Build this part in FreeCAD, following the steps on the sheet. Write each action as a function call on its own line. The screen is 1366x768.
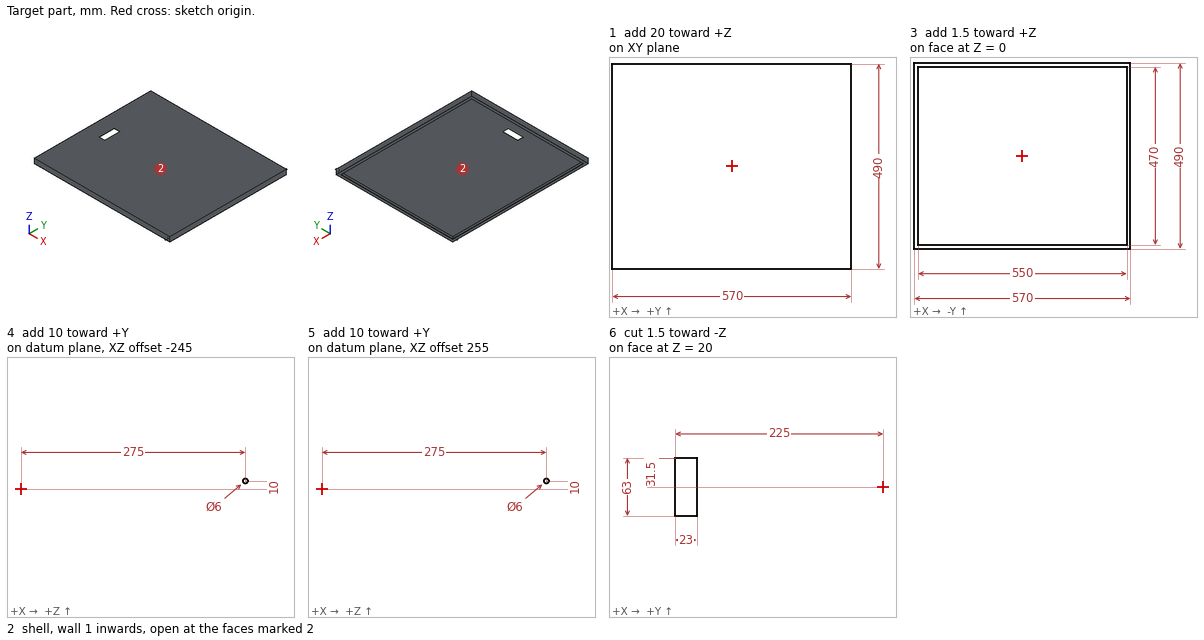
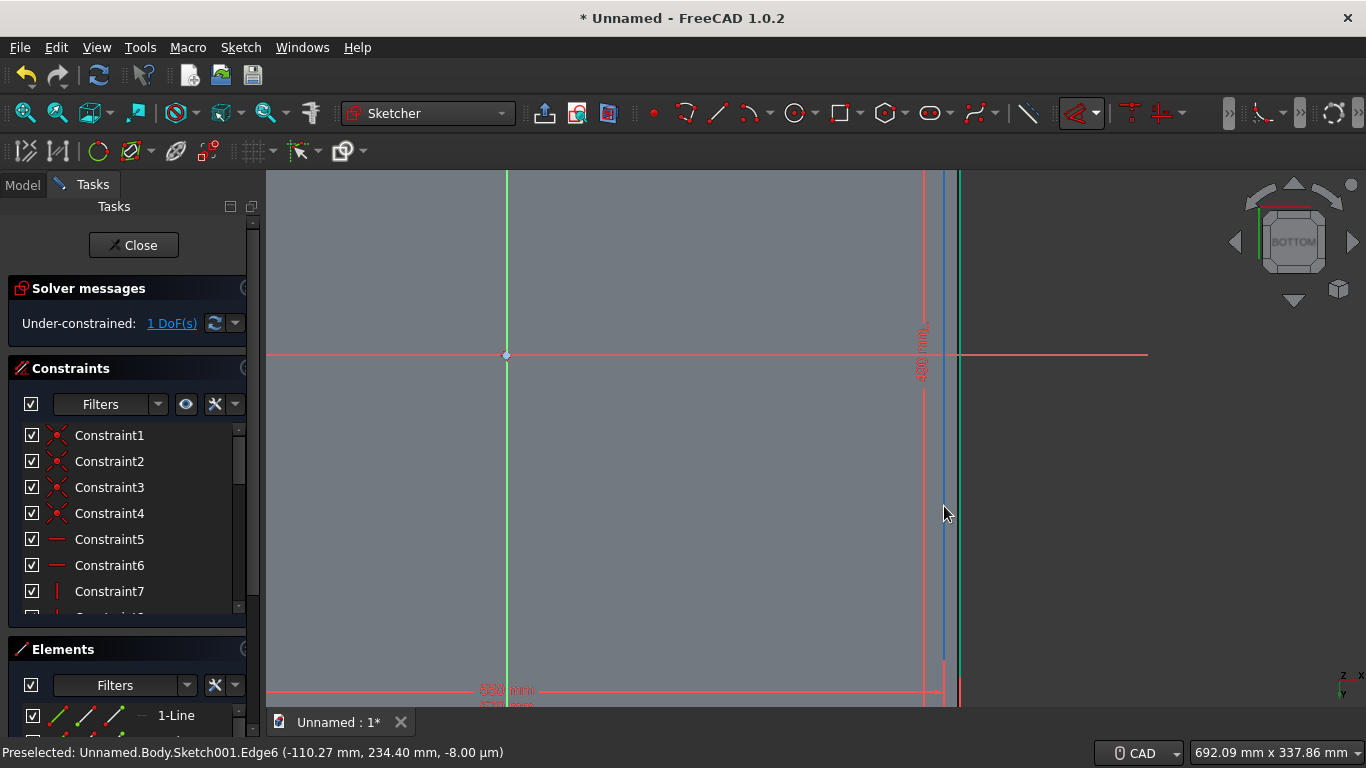
click(944, 504)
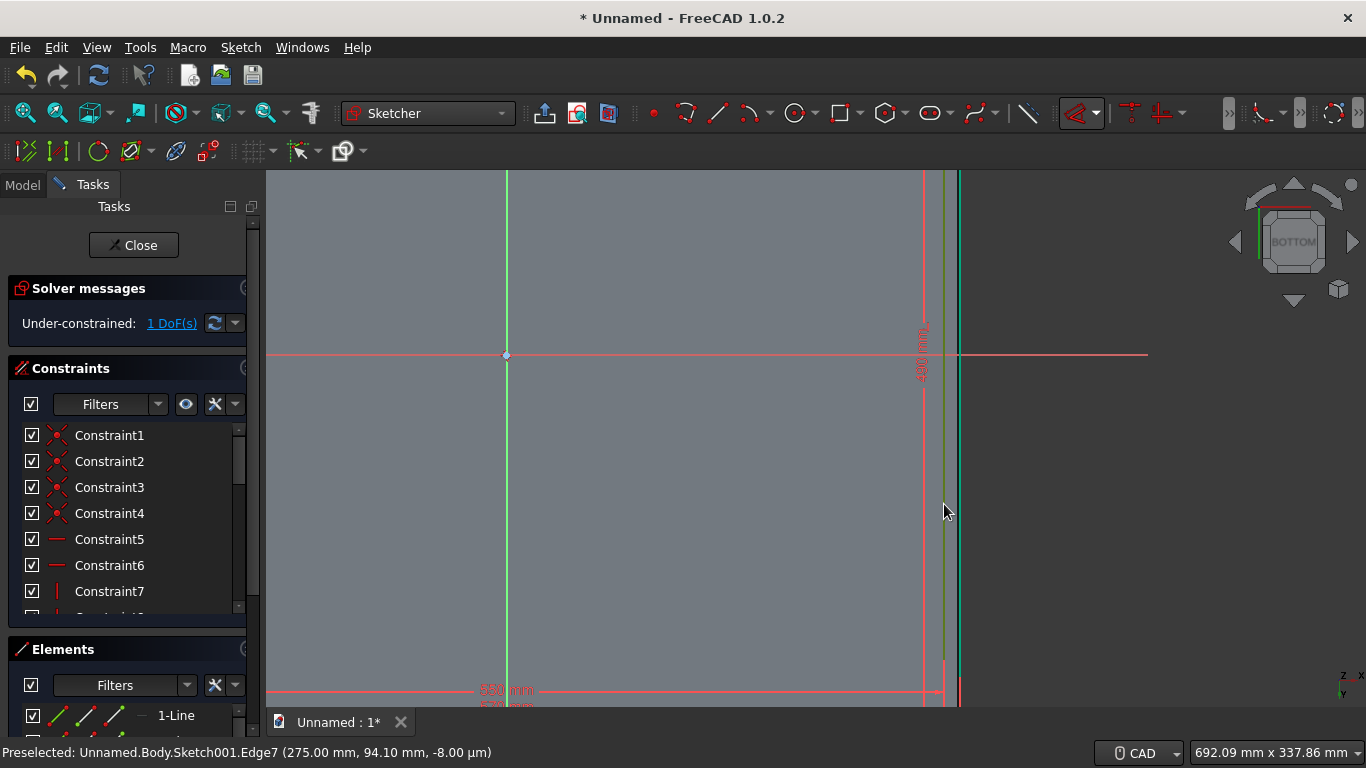
click(1098, 114)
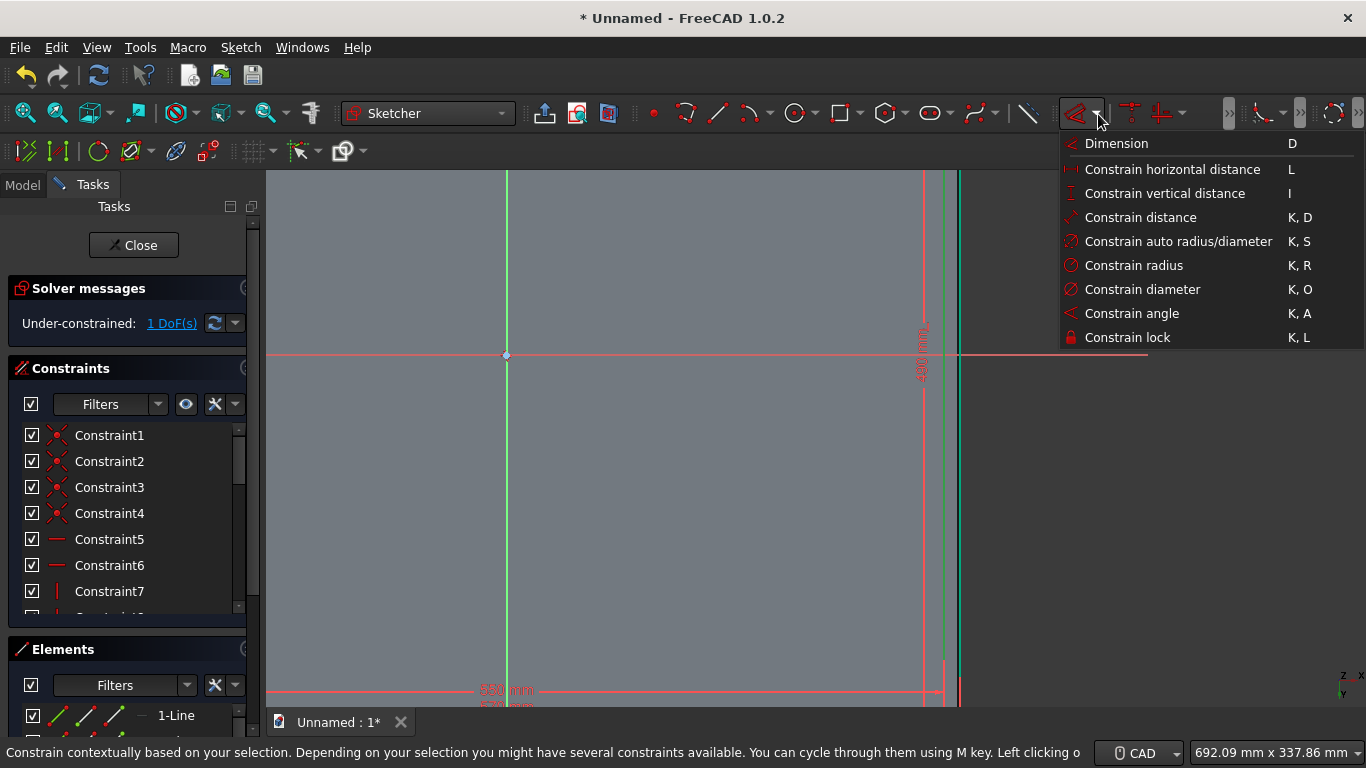
click(1212, 193)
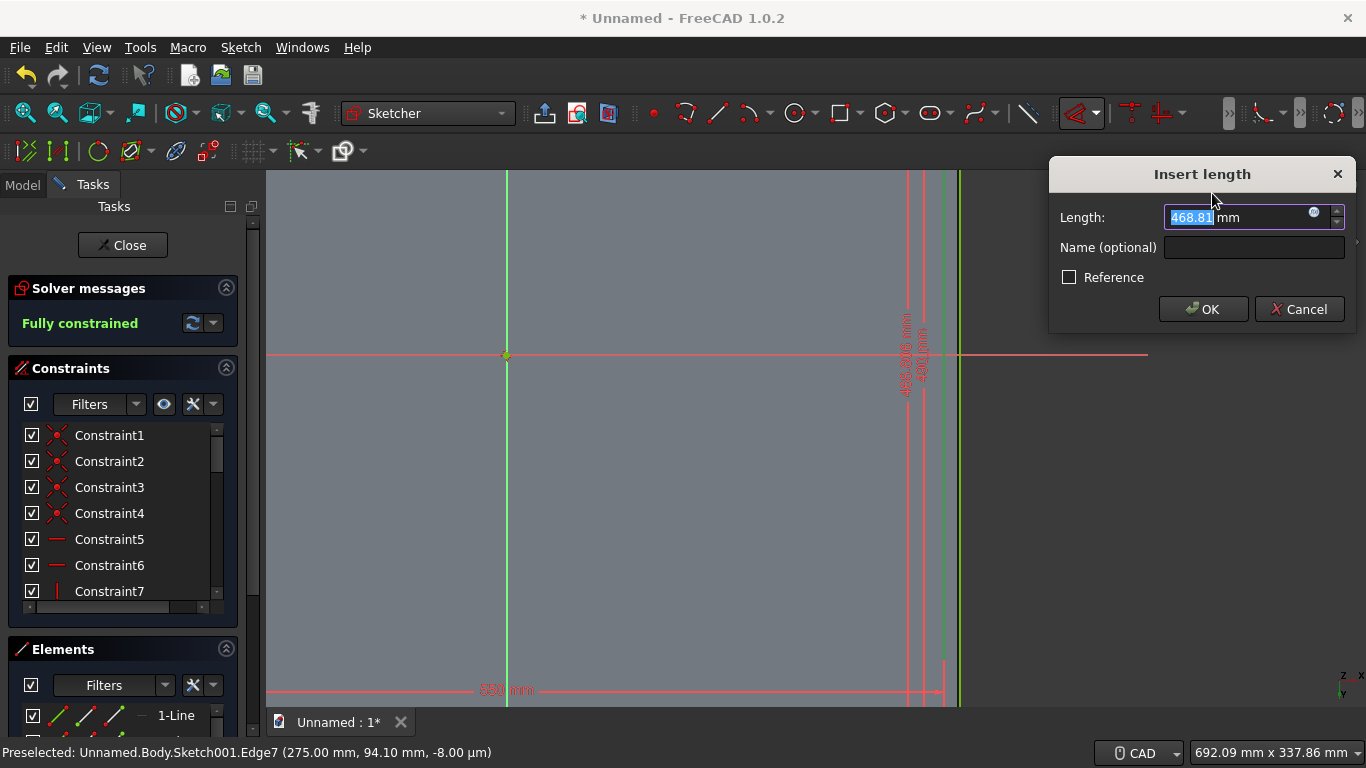
text(470)
key(Return)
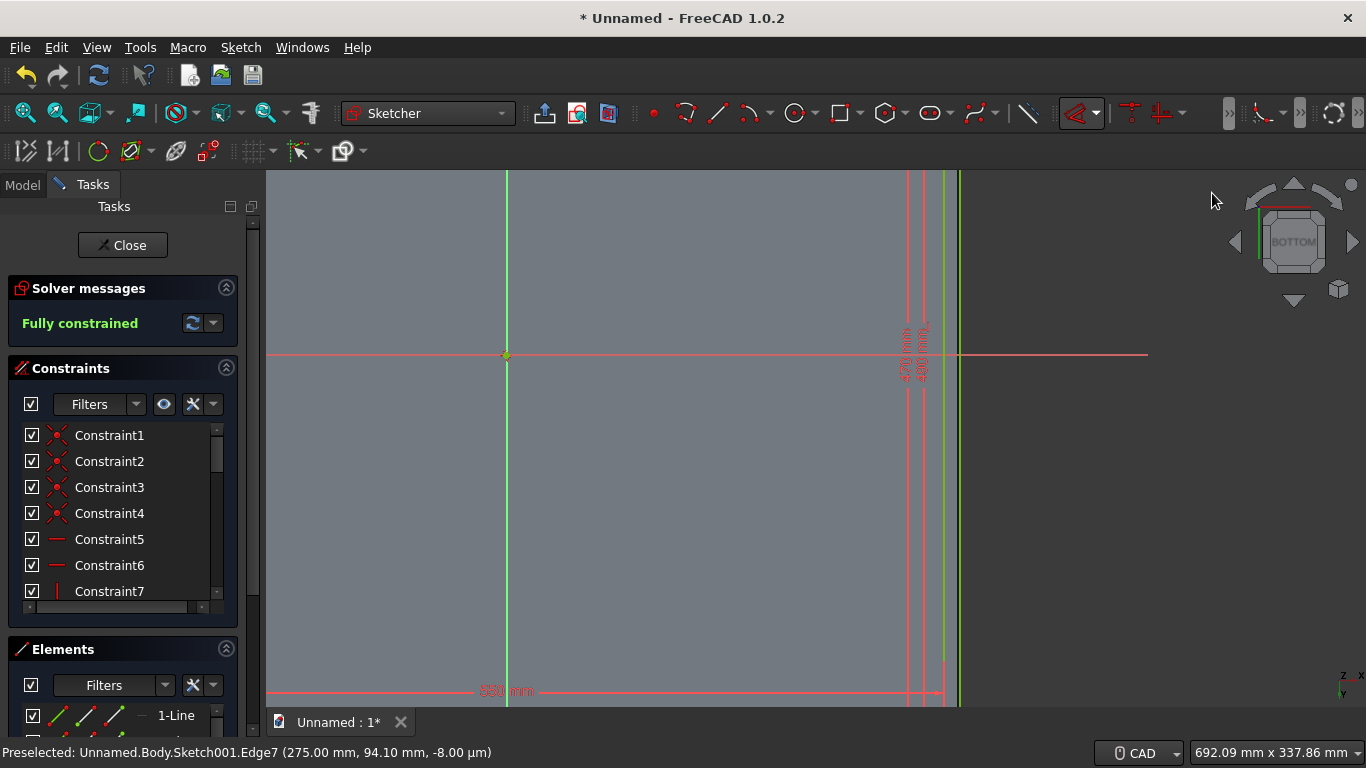
click(123, 245)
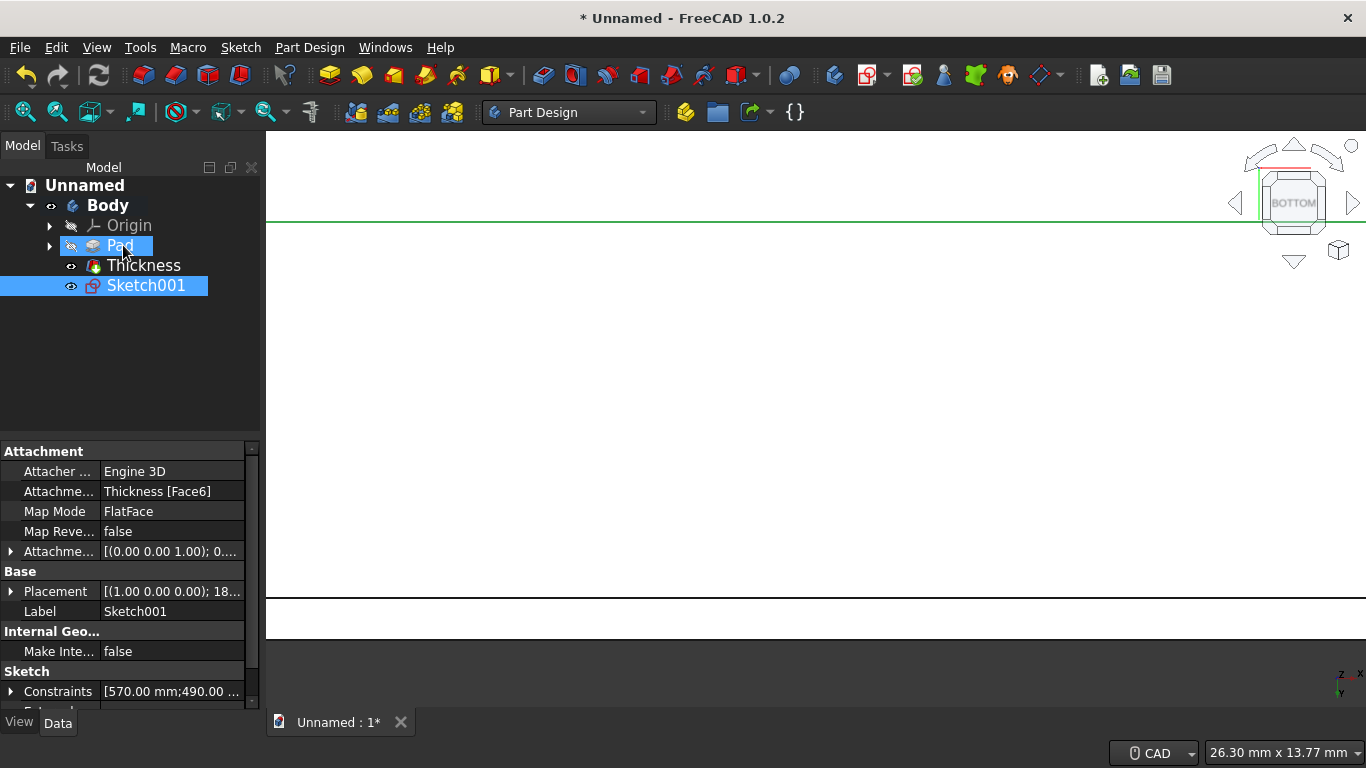
click(330, 76)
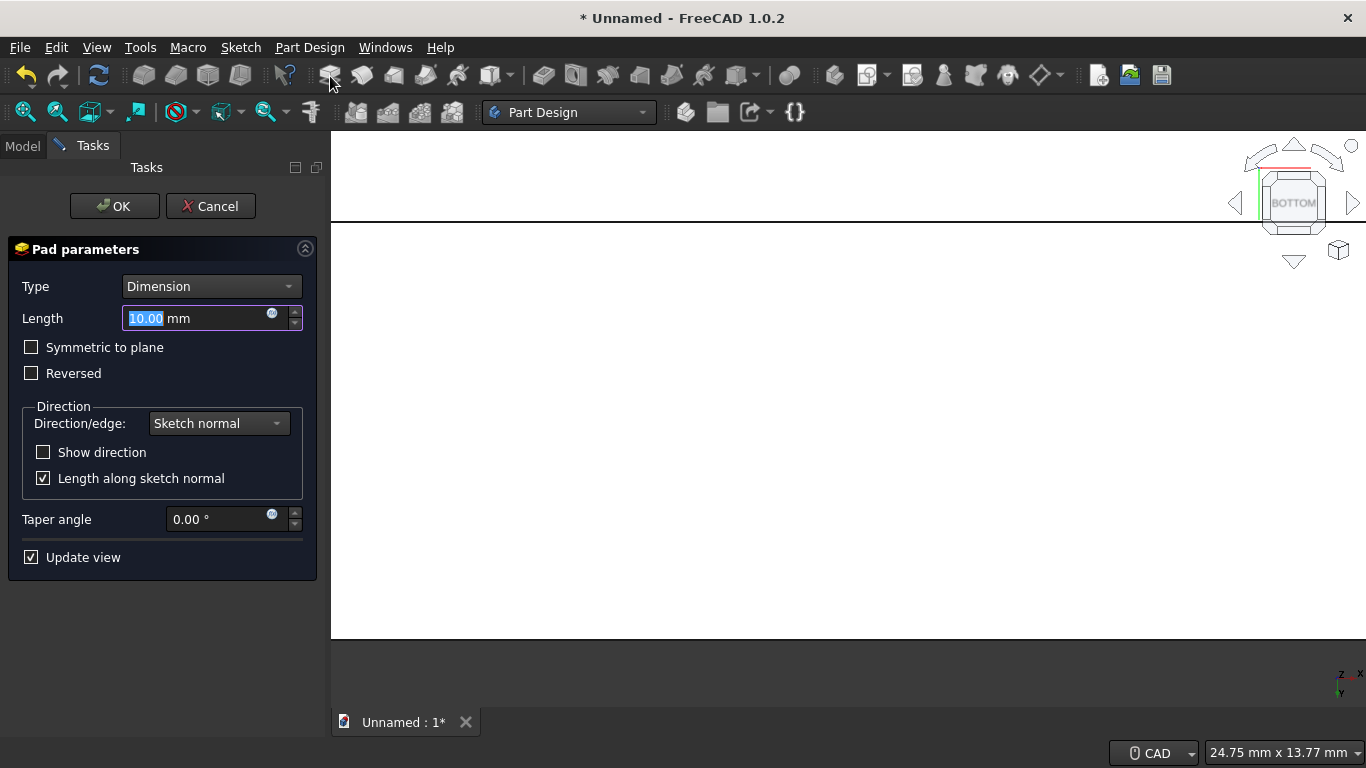
text(1.5)
key(Tab)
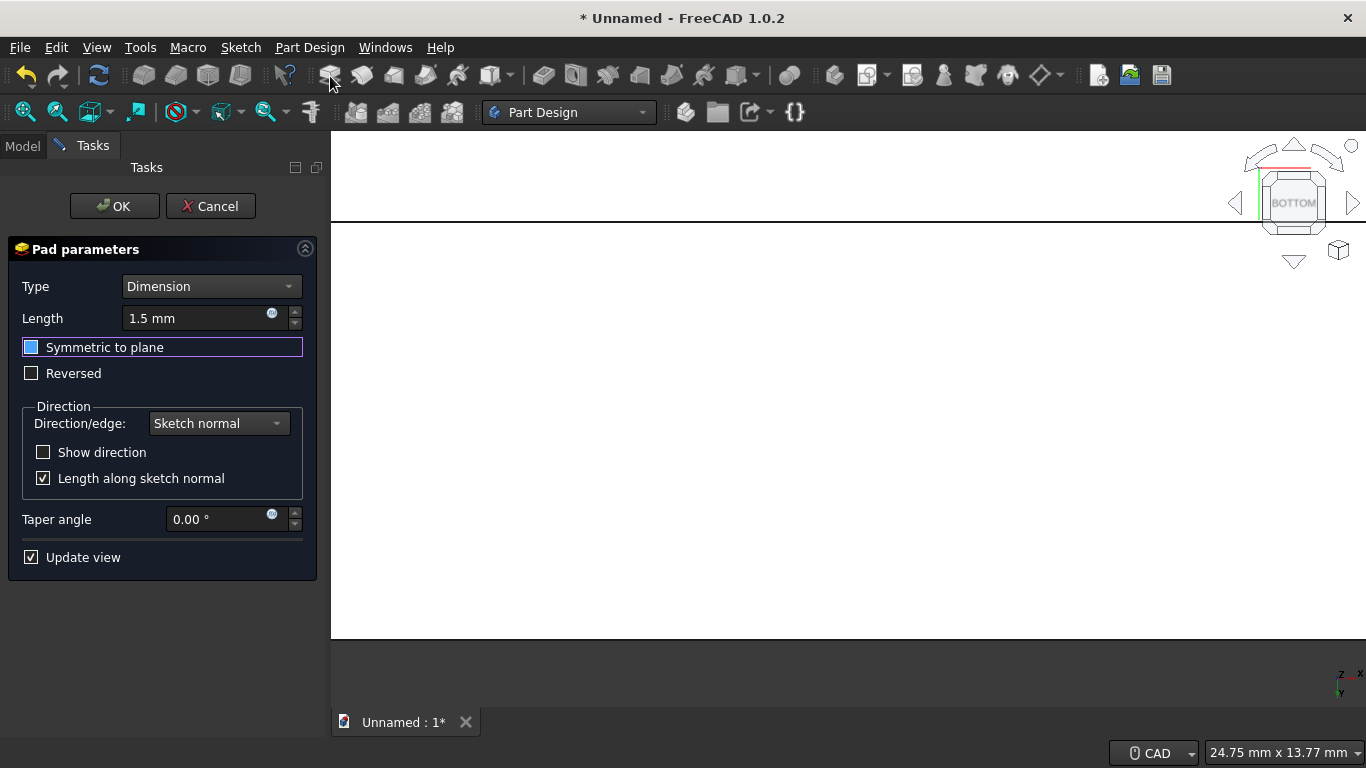
click(30, 373)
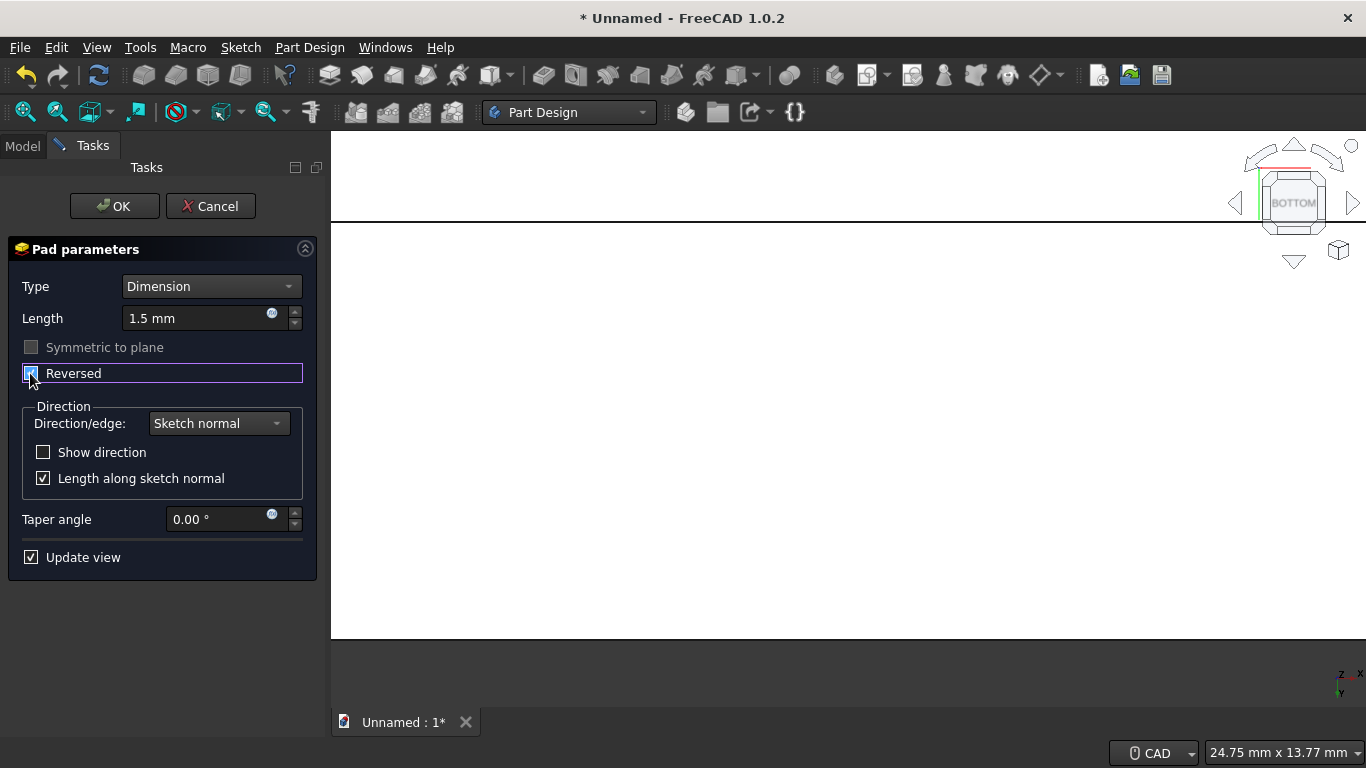
click(115, 206)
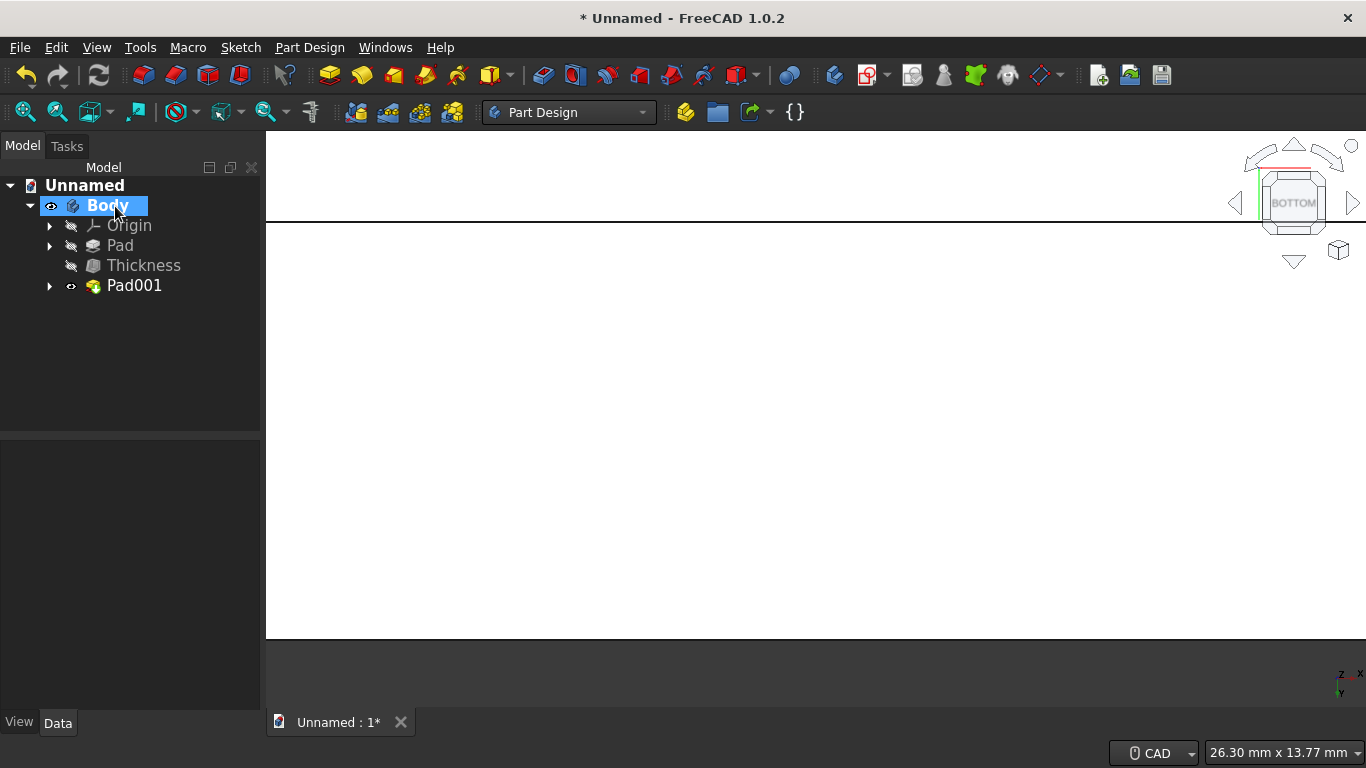
key(v)
key(f)